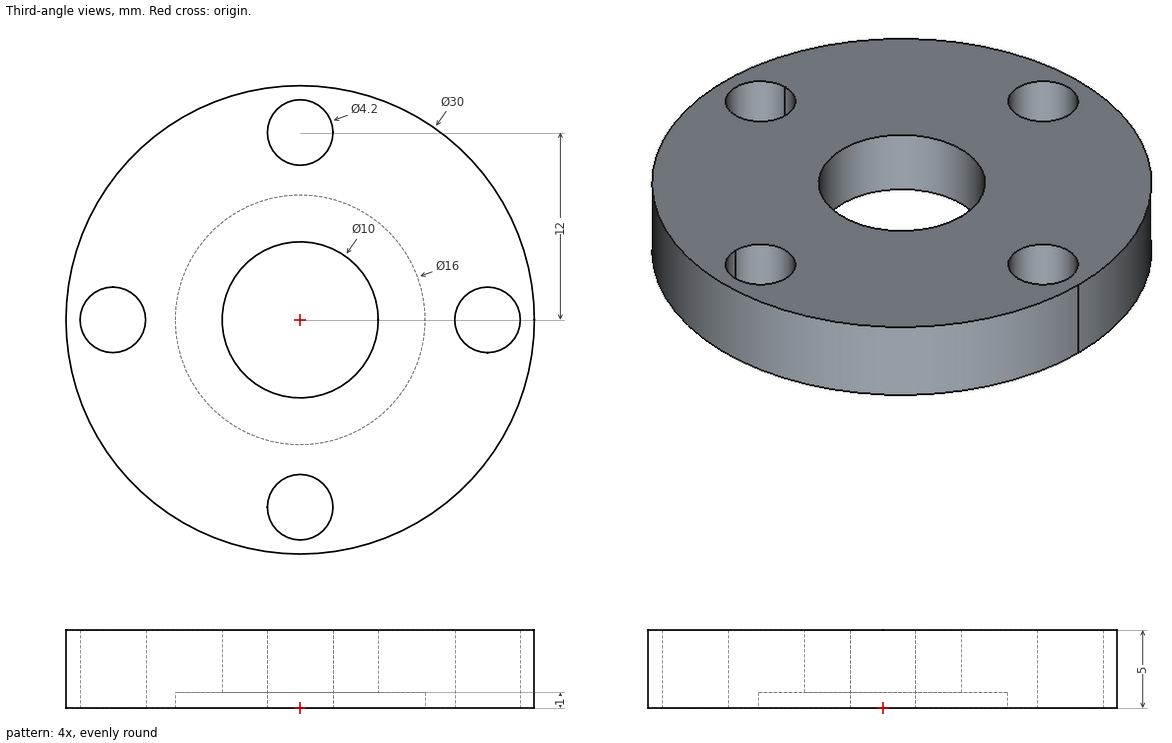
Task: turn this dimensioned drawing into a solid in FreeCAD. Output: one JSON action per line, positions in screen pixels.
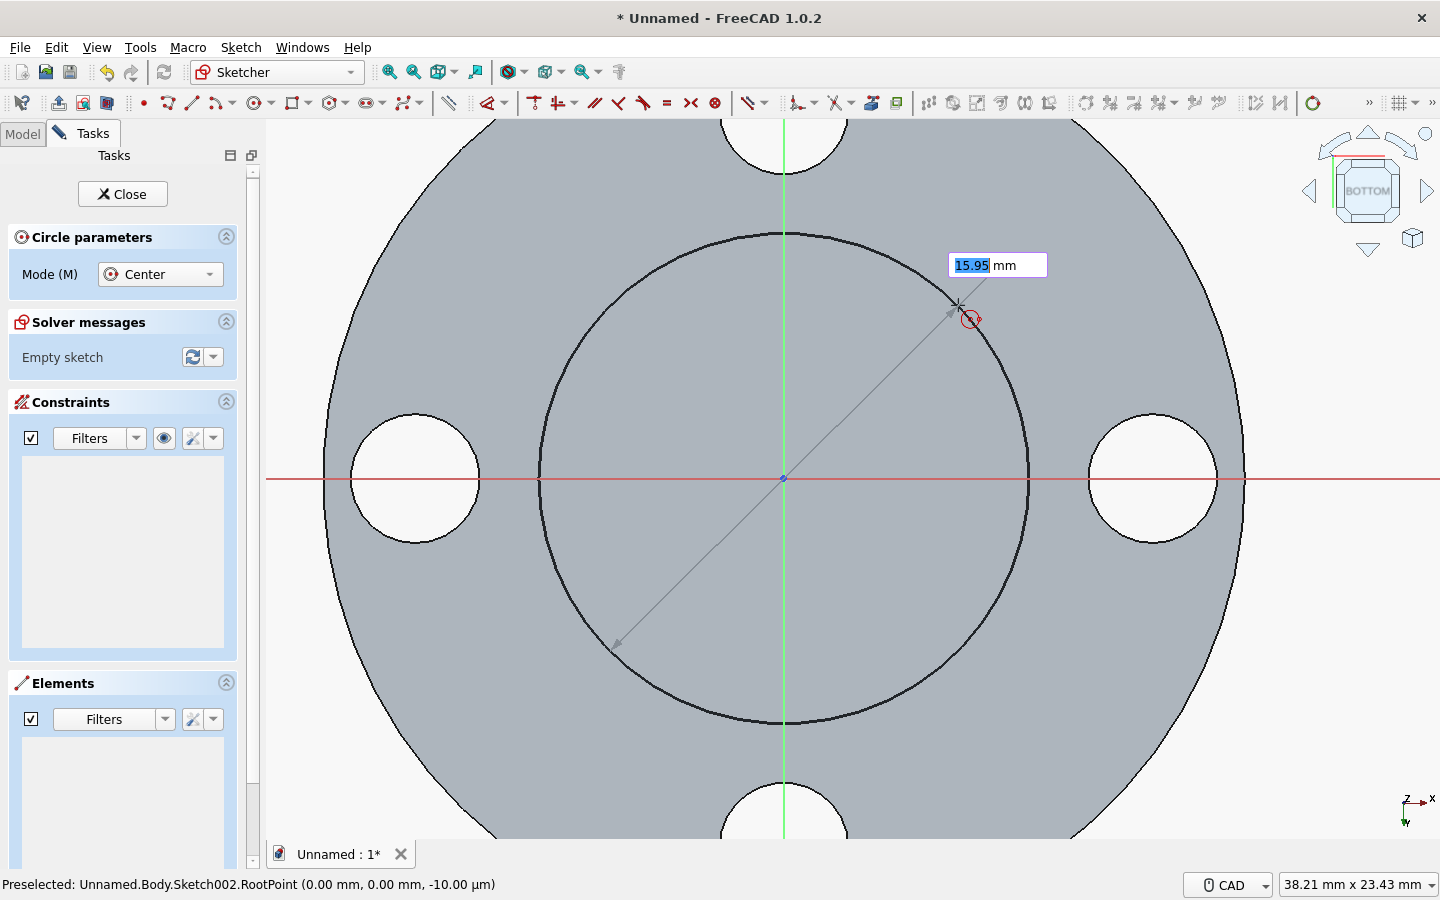
{"action": "type", "text": "16"}
{"action": "key", "text": "Return"}
{"action": "key", "text": "Escape"}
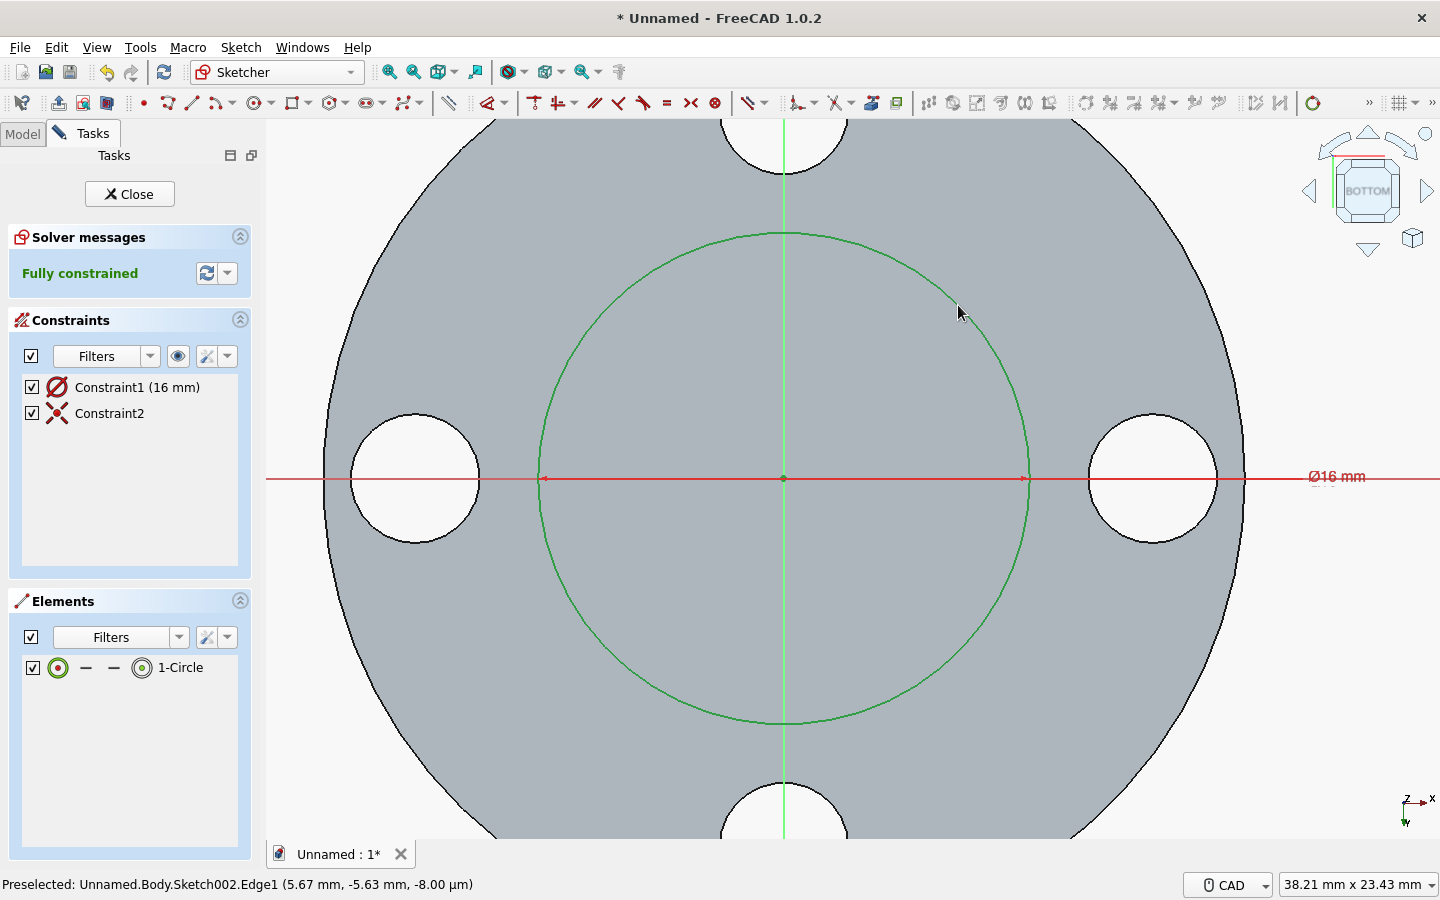
{"action": "left_click", "coordinate": [130, 194]}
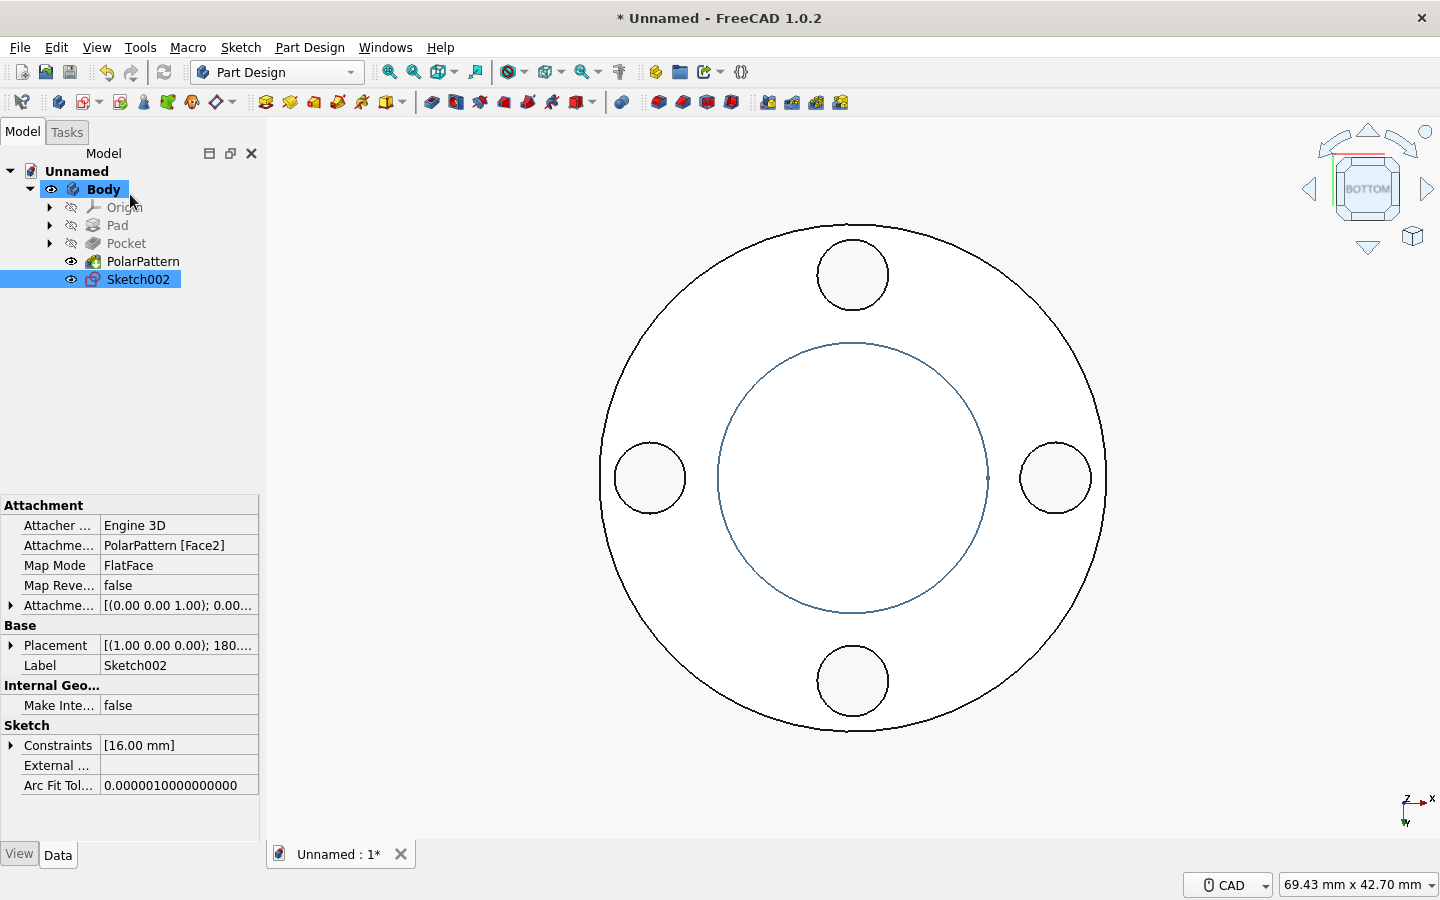
{"action": "left_click", "coordinate": [432, 102]}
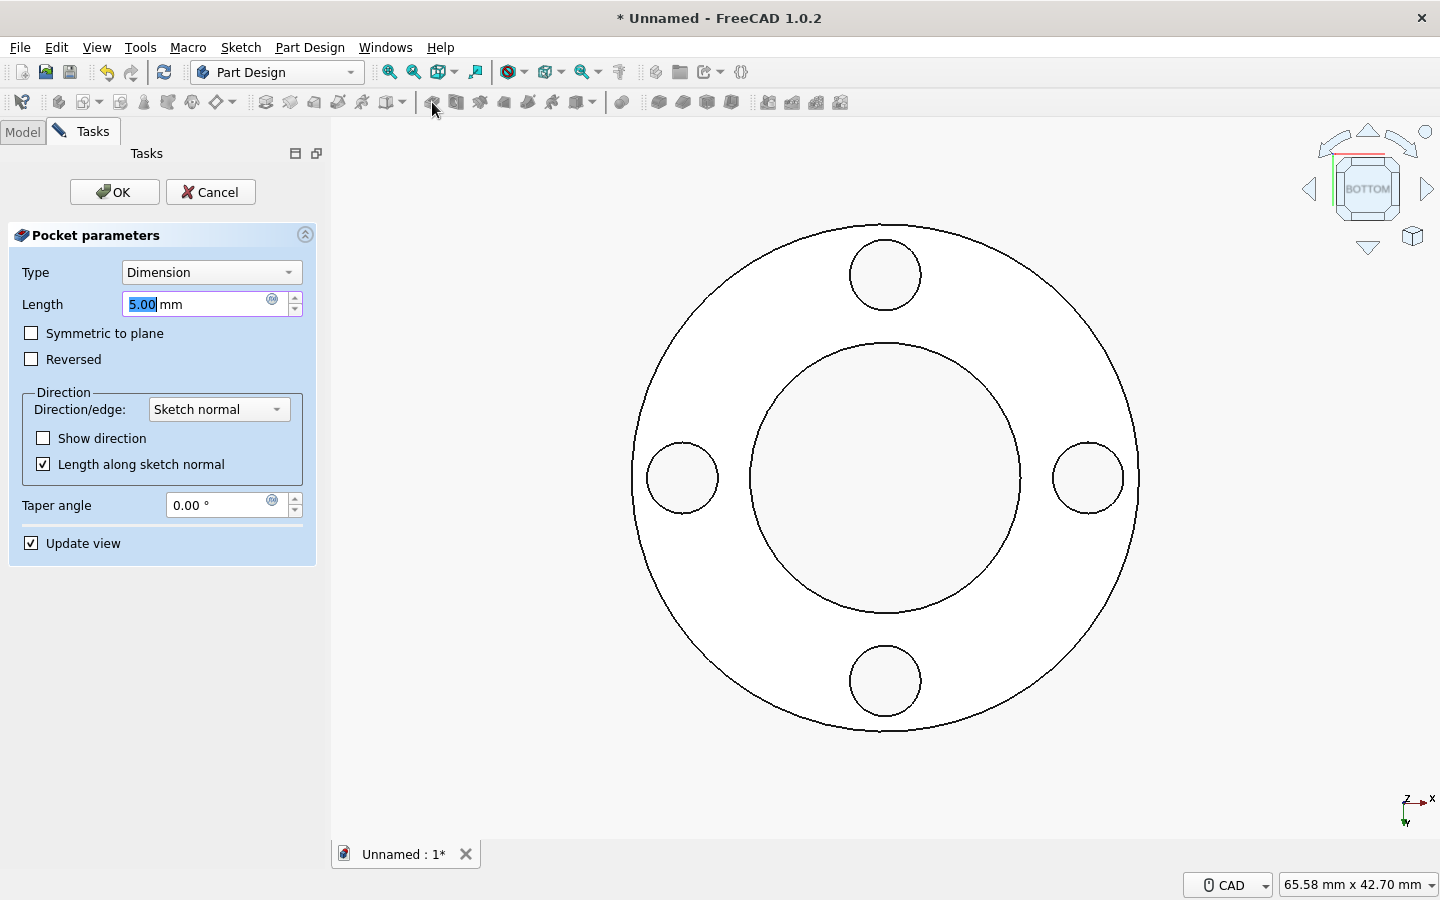
{"action": "type", "text": "1"}
{"action": "key", "text": "Tab"}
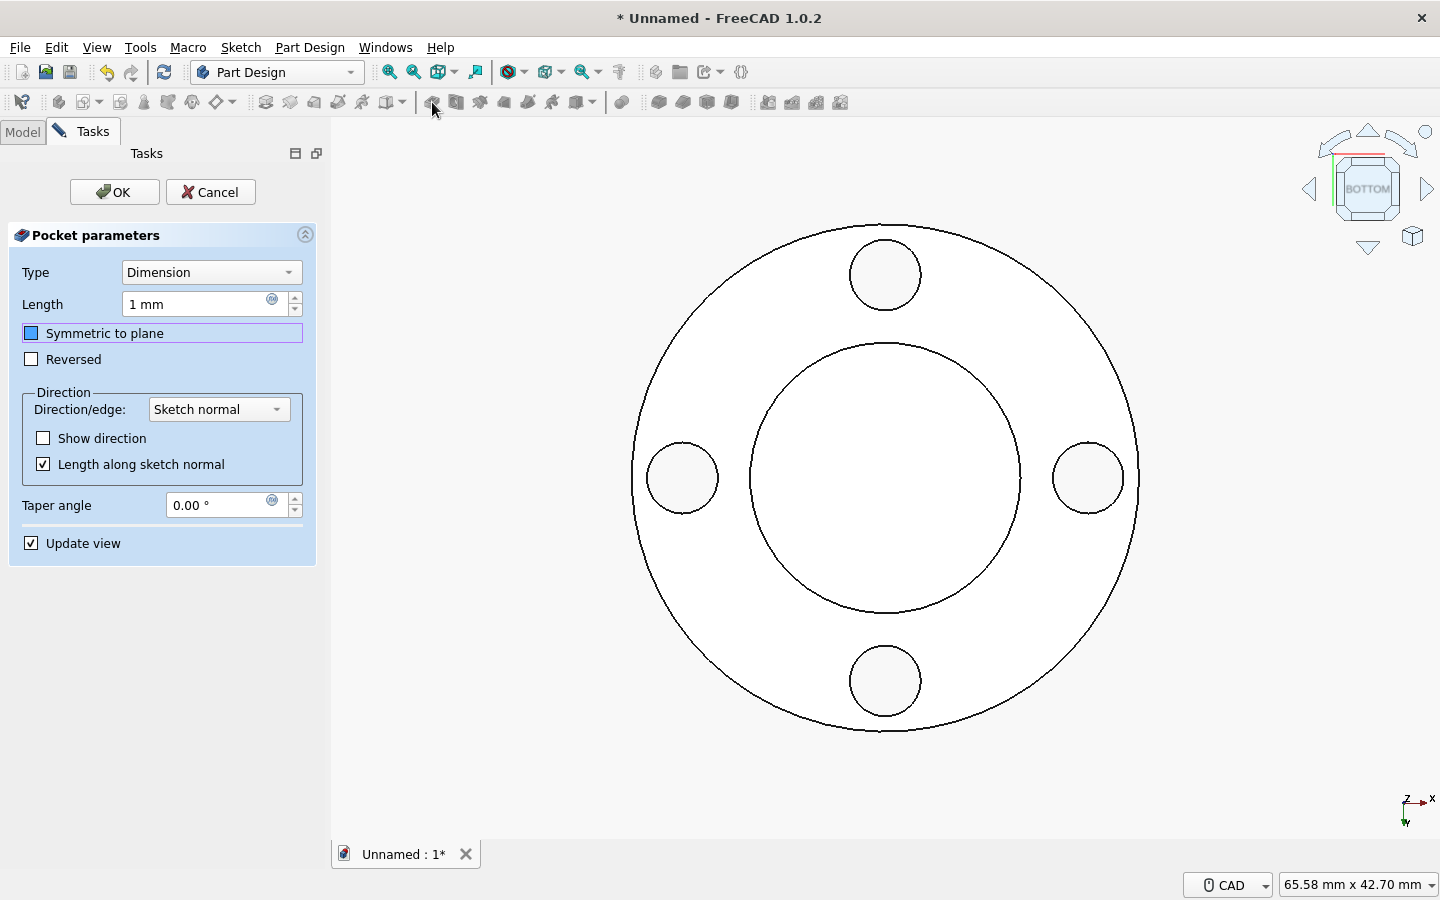
{"action": "left_click", "coordinate": [115, 192]}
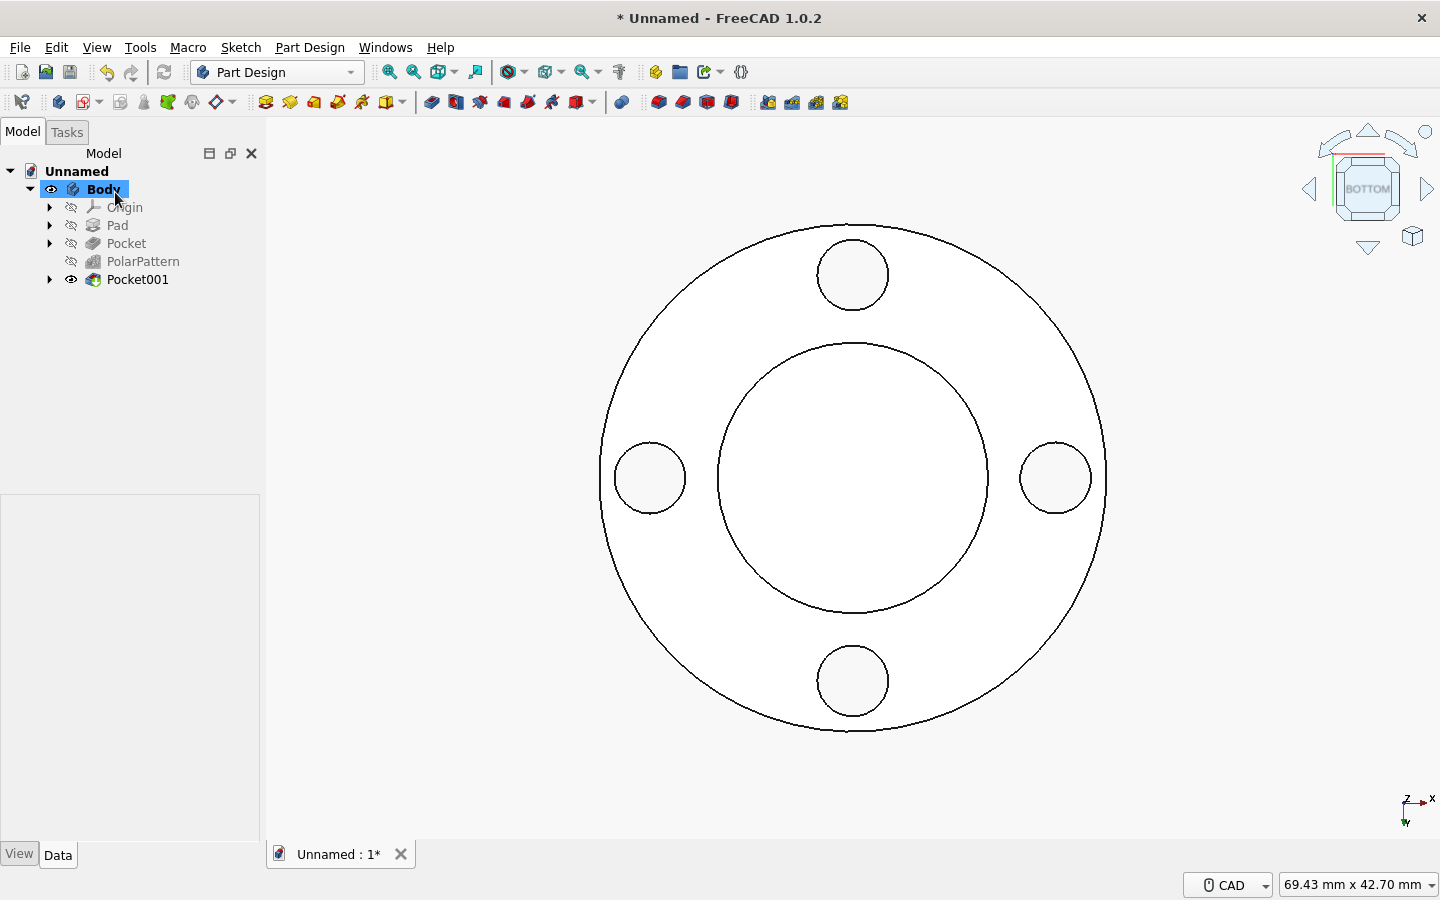
{"action": "key", "text": "0"}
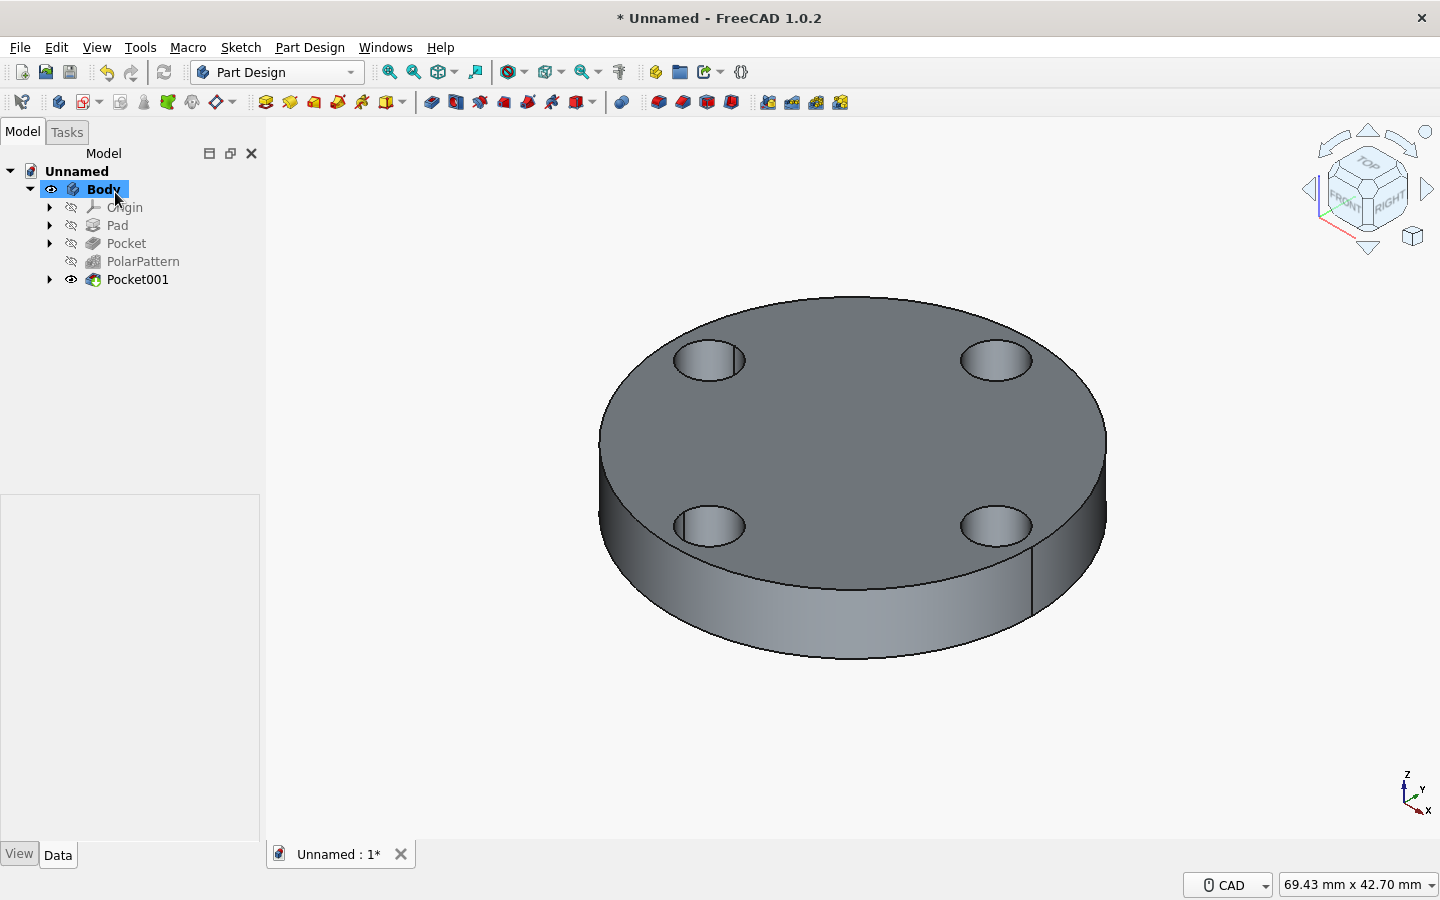
{"action": "left_click", "coordinate": [853, 442]}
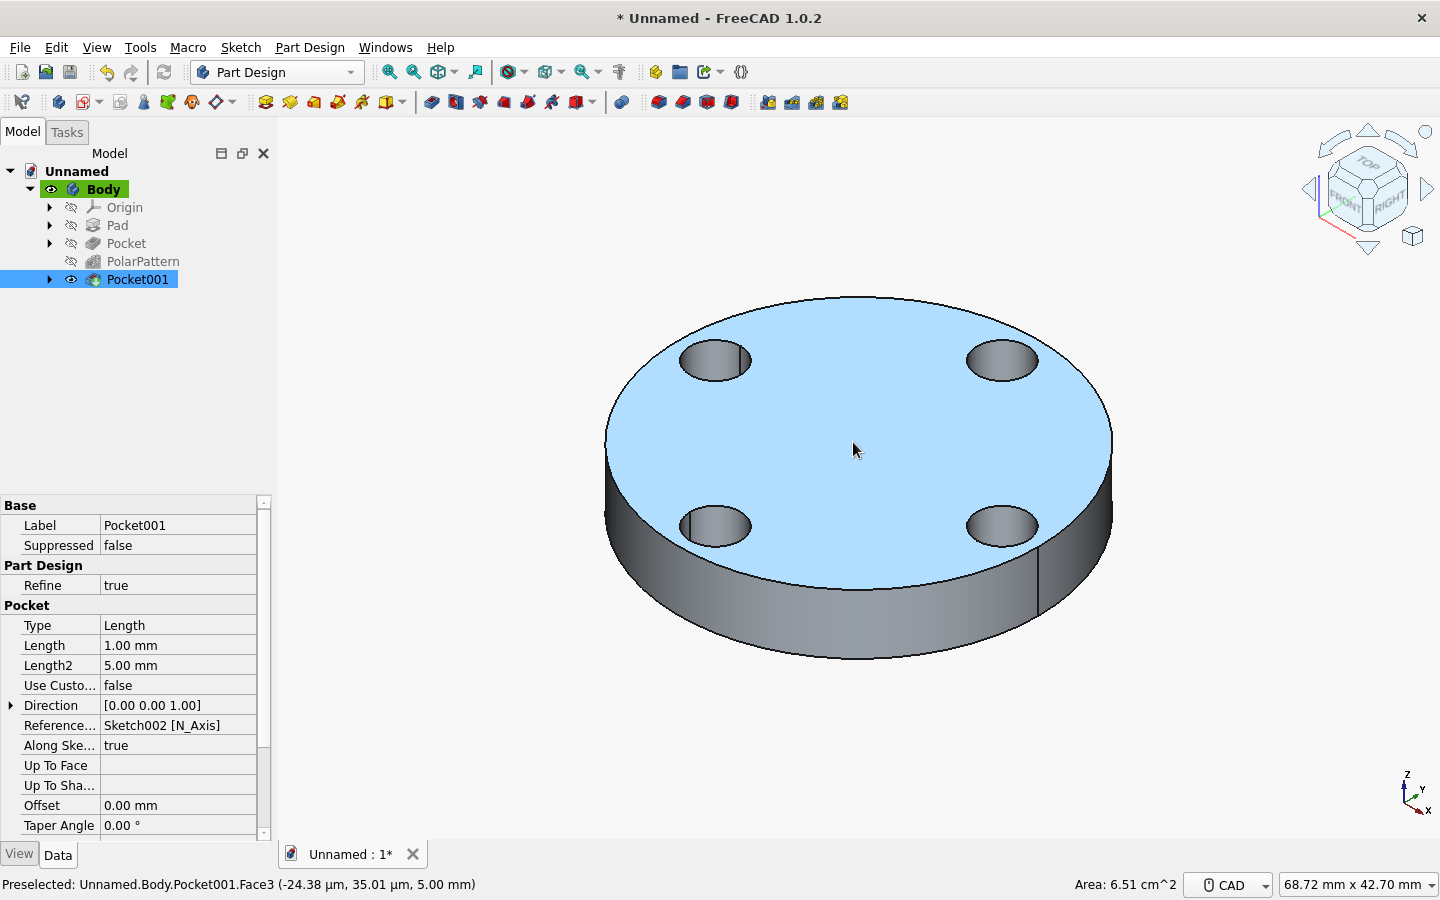
{"action": "left_click", "coordinate": [84, 102]}